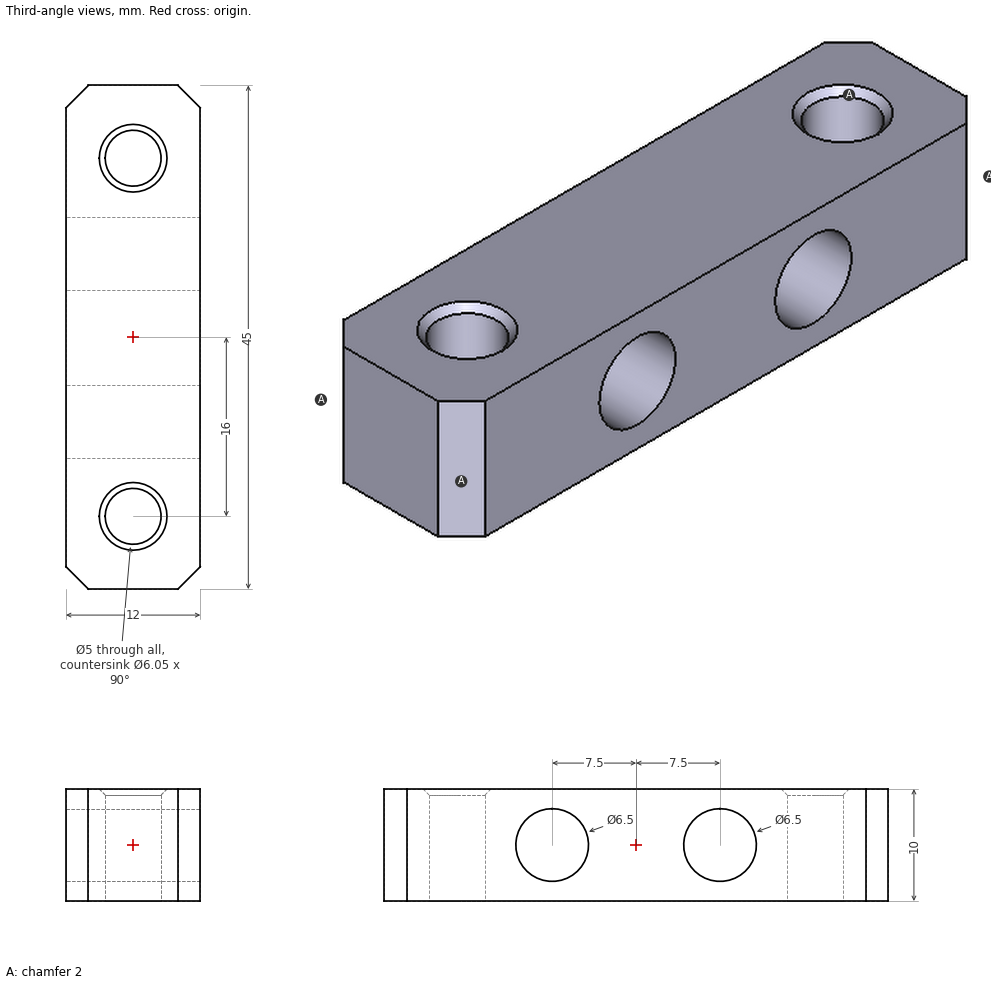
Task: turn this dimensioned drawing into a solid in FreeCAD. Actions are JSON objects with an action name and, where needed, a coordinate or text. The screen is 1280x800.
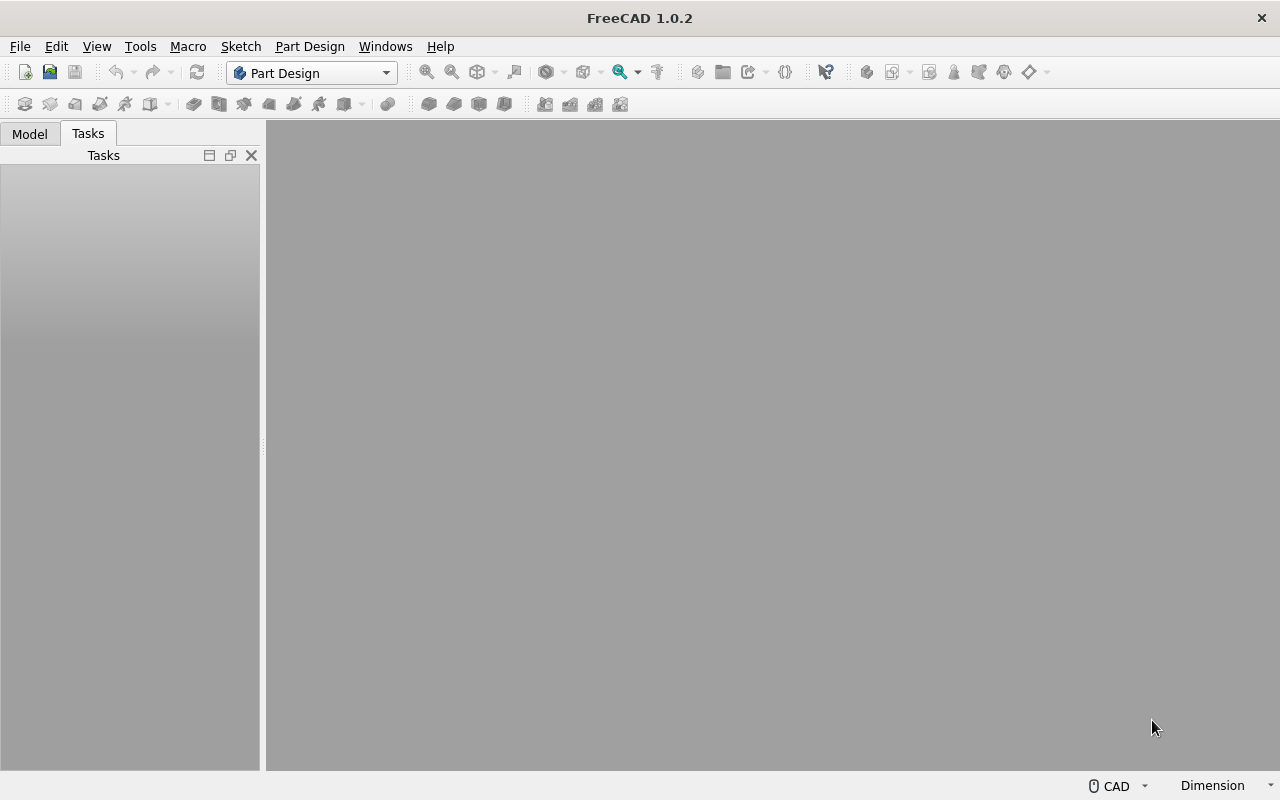
{"action": "left_click", "coordinate": [25, 72]}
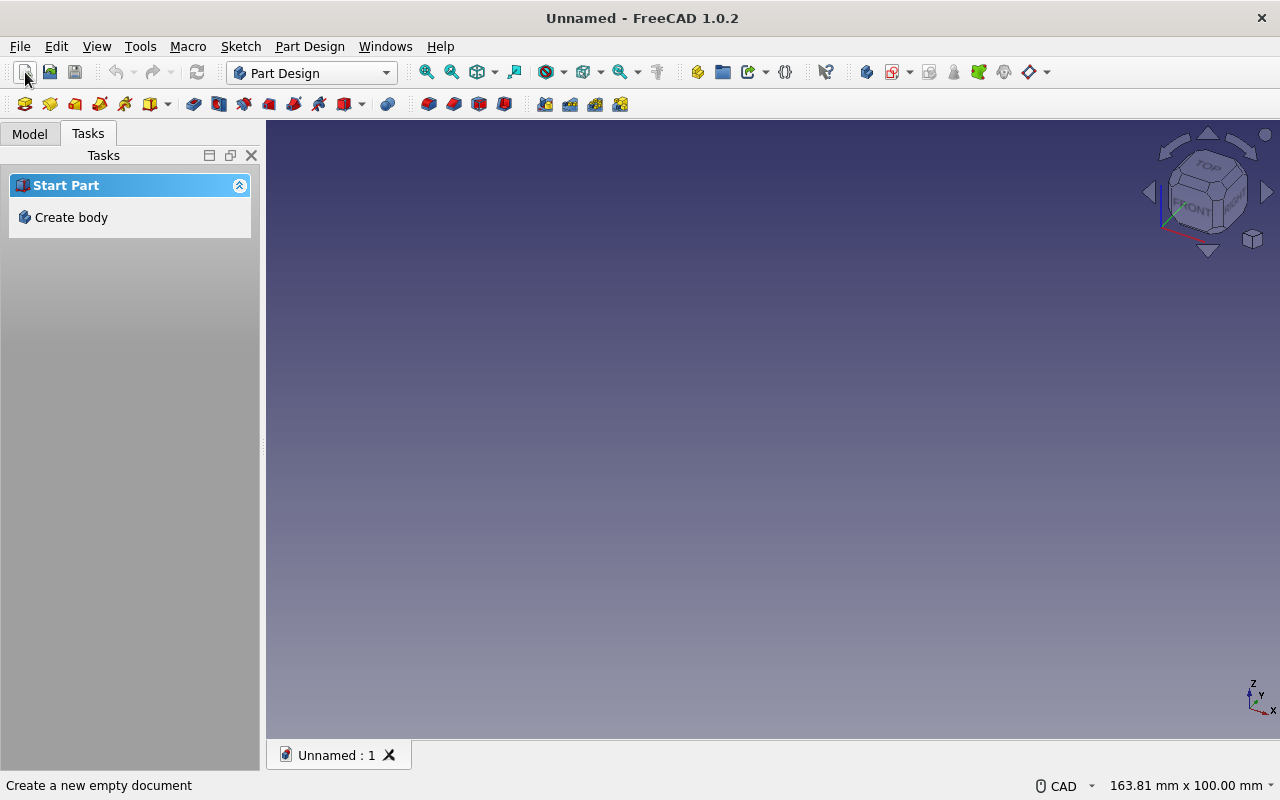
{"action": "left_click", "coordinate": [892, 72]}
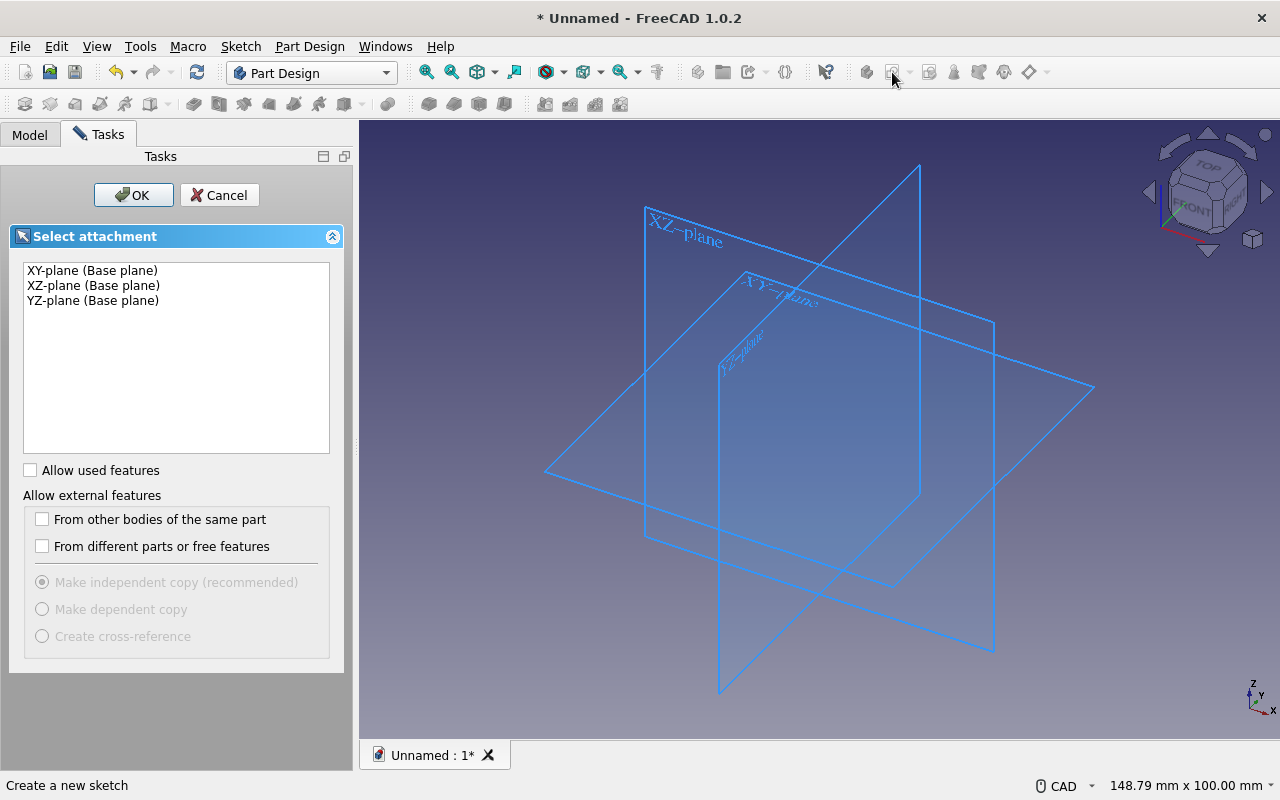
{"action": "left_click", "coordinate": [84, 270]}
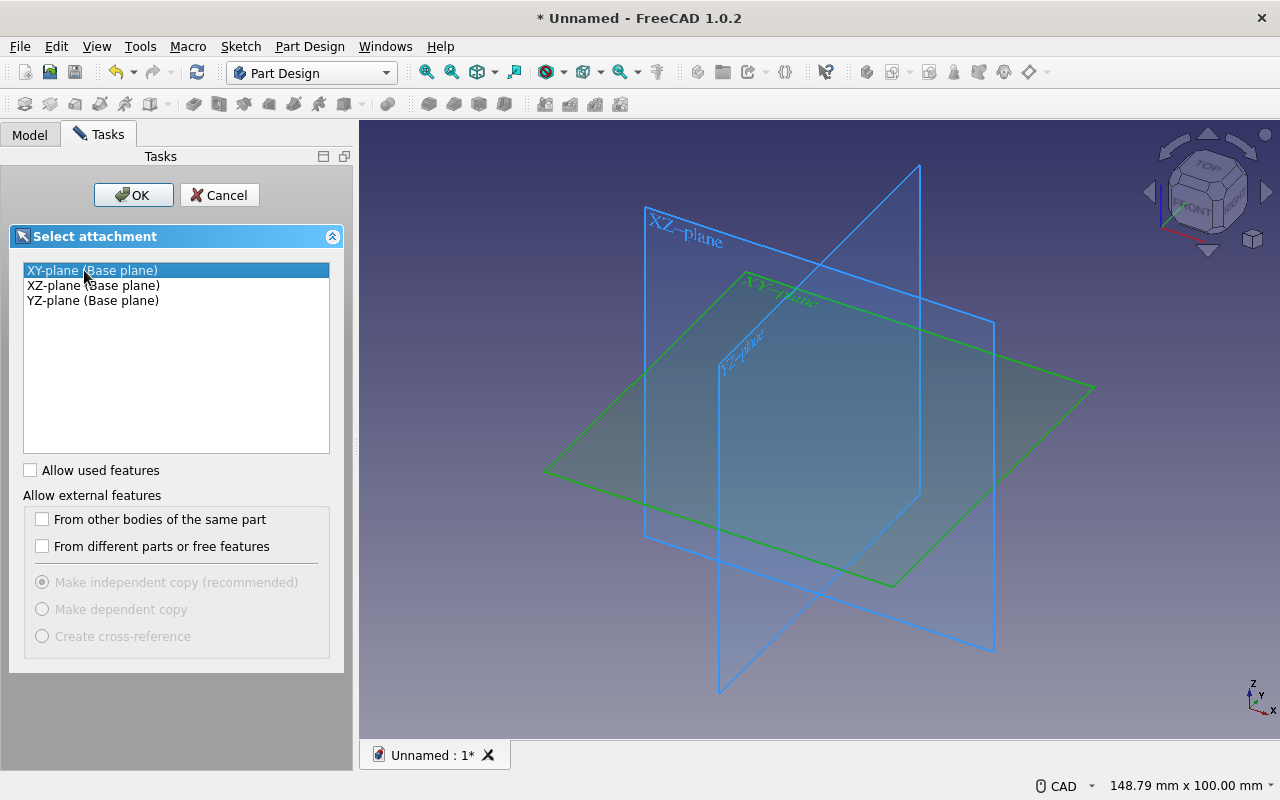
{"action": "left_click", "coordinate": [134, 195]}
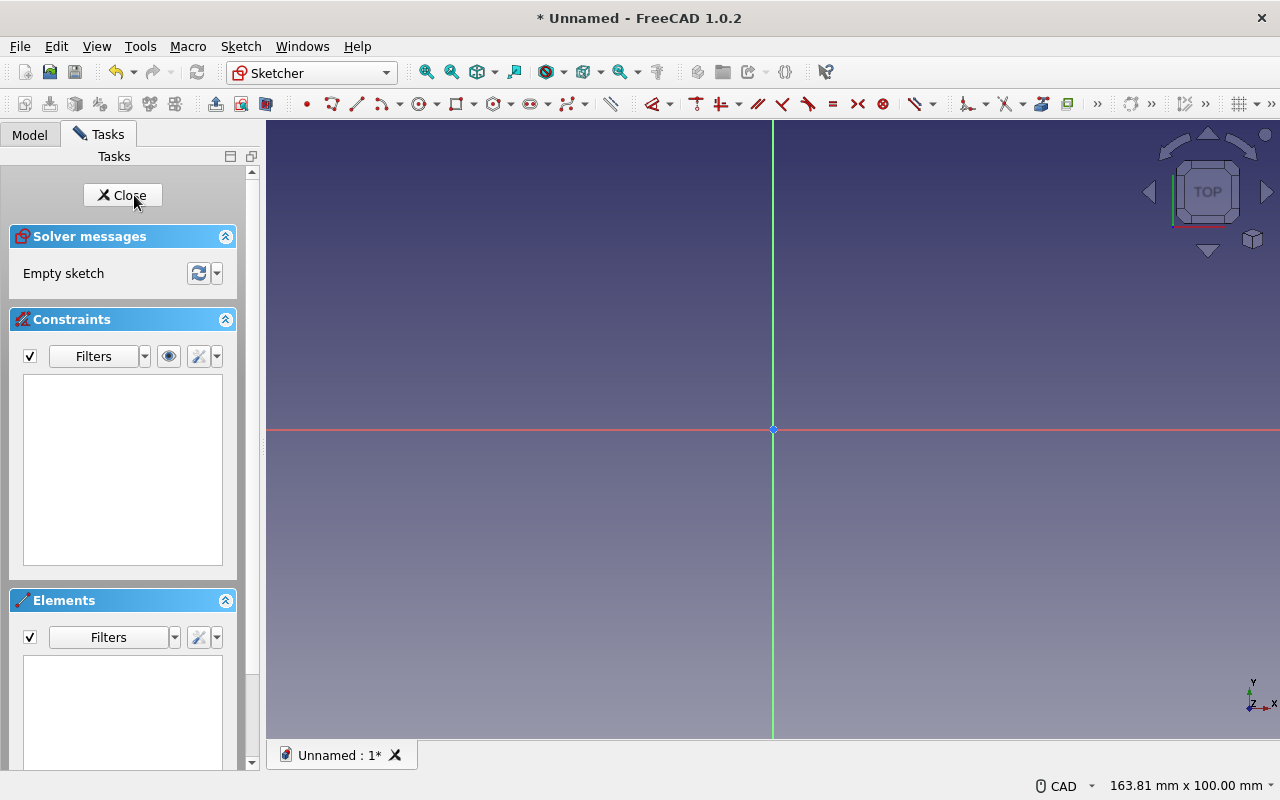
{"action": "scroll", "coordinate": [912, 429], "scroll_direction": "up", "scroll_amount": 2}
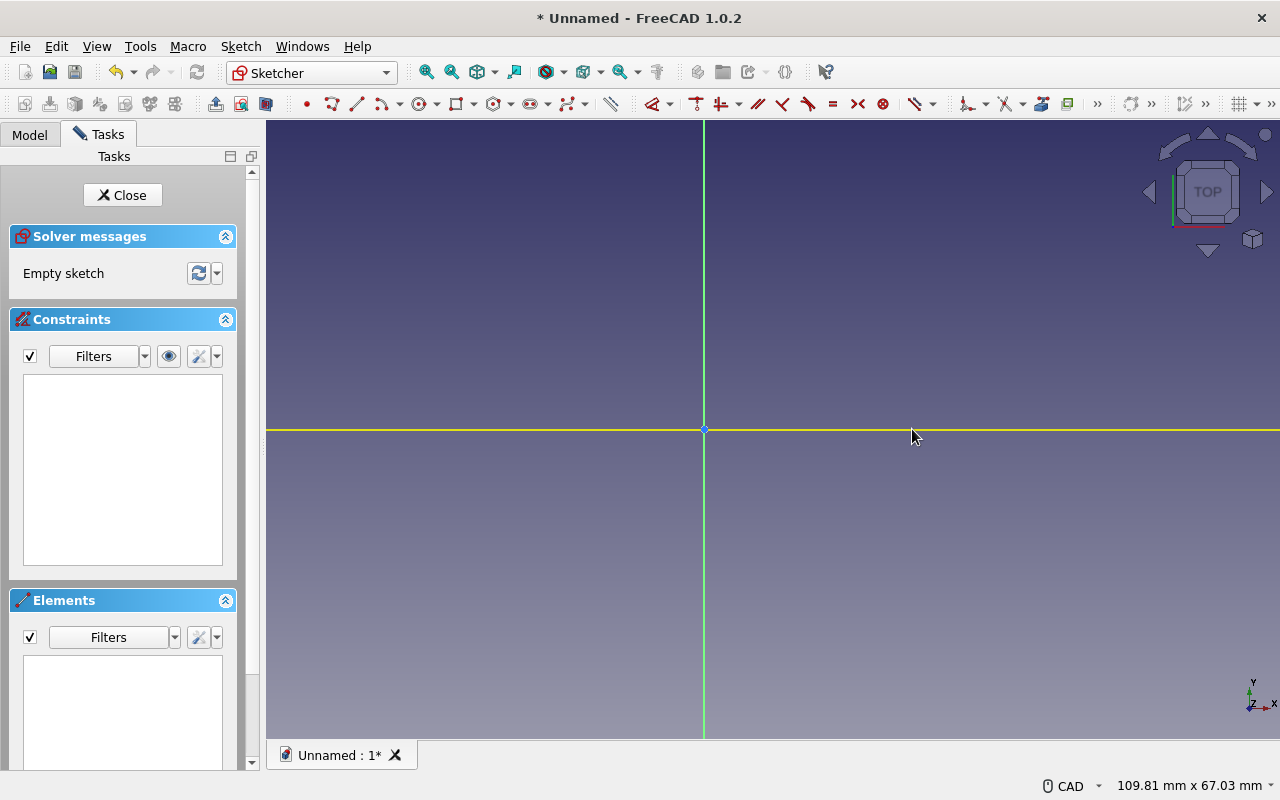
{"action": "key", "text": "g v"}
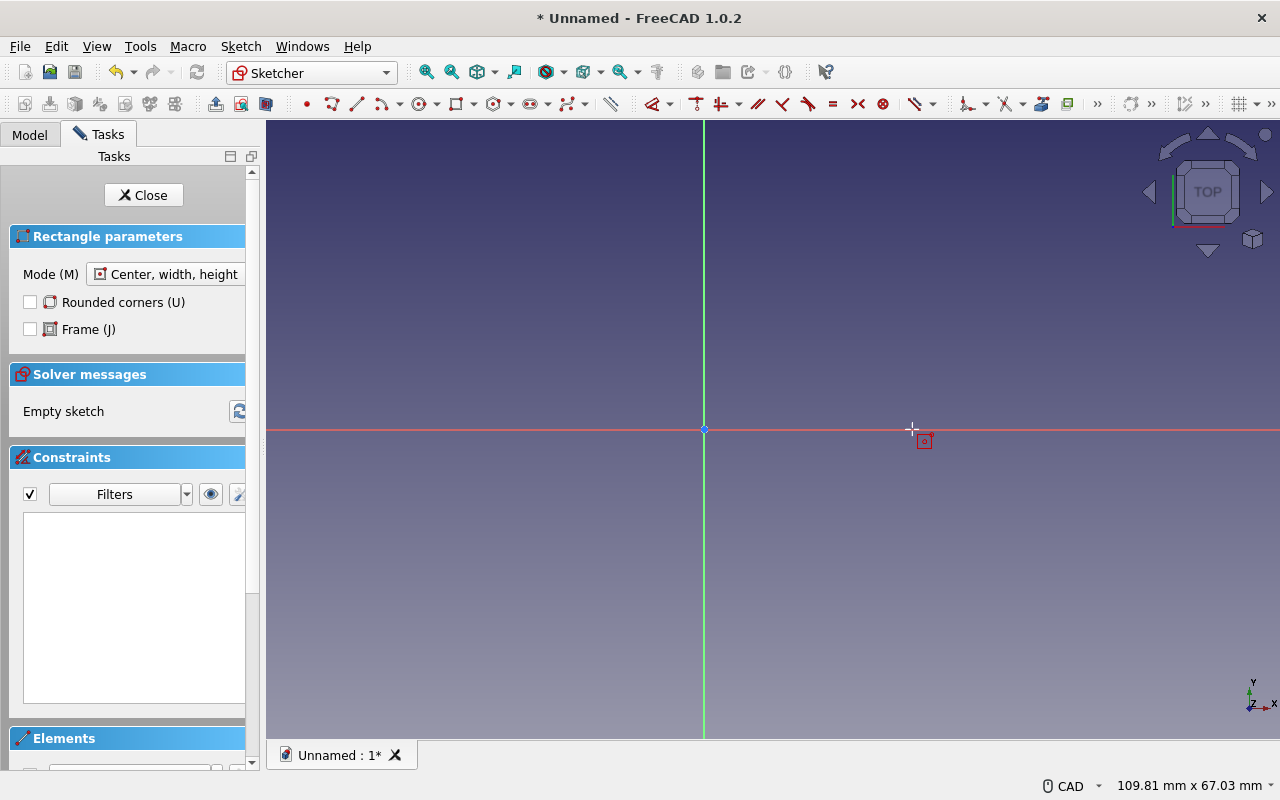
{"action": "left_click", "coordinate": [704, 430]}
{"action": "mouse_move", "coordinate": [760, 222]}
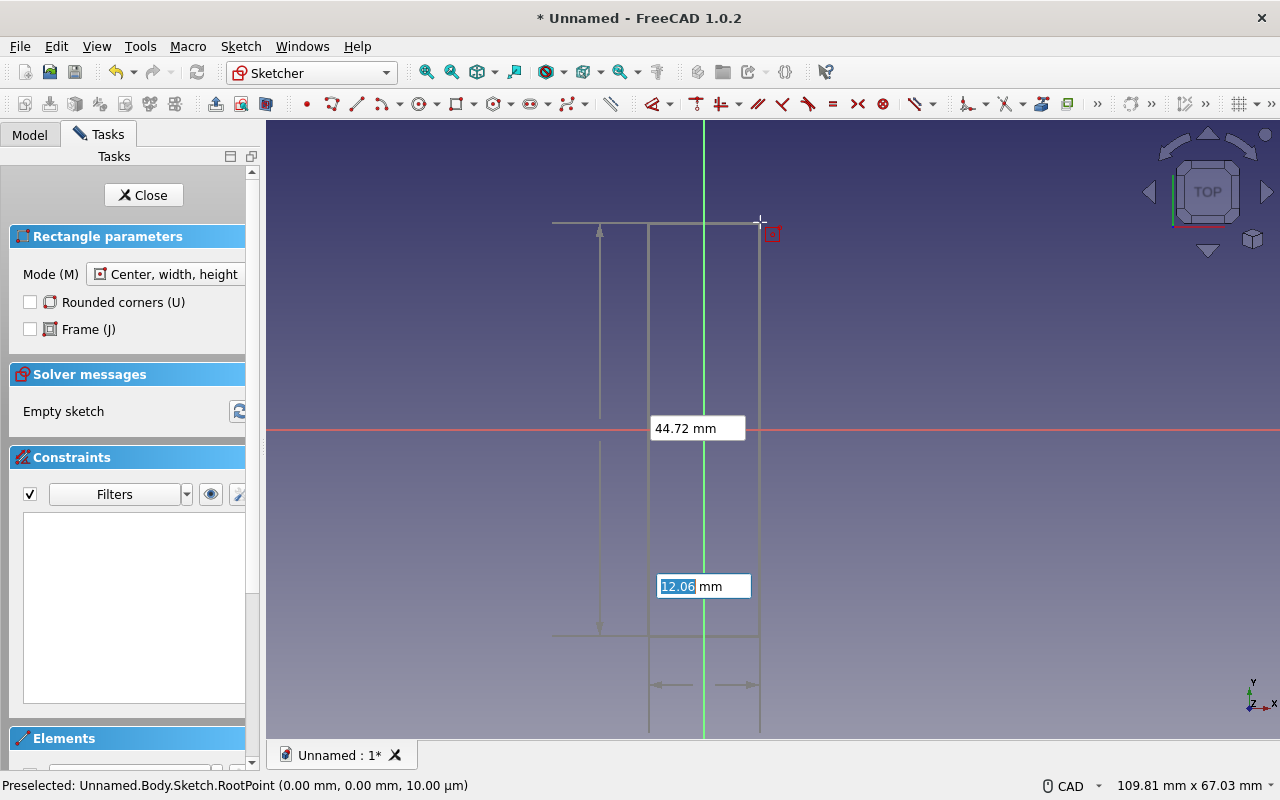
{"action": "type", "text": "12"}
{"action": "key", "text": "Tab"}
{"action": "type", "text": "45"}
{"action": "key", "text": "Return"}
{"action": "key", "text": "Escape"}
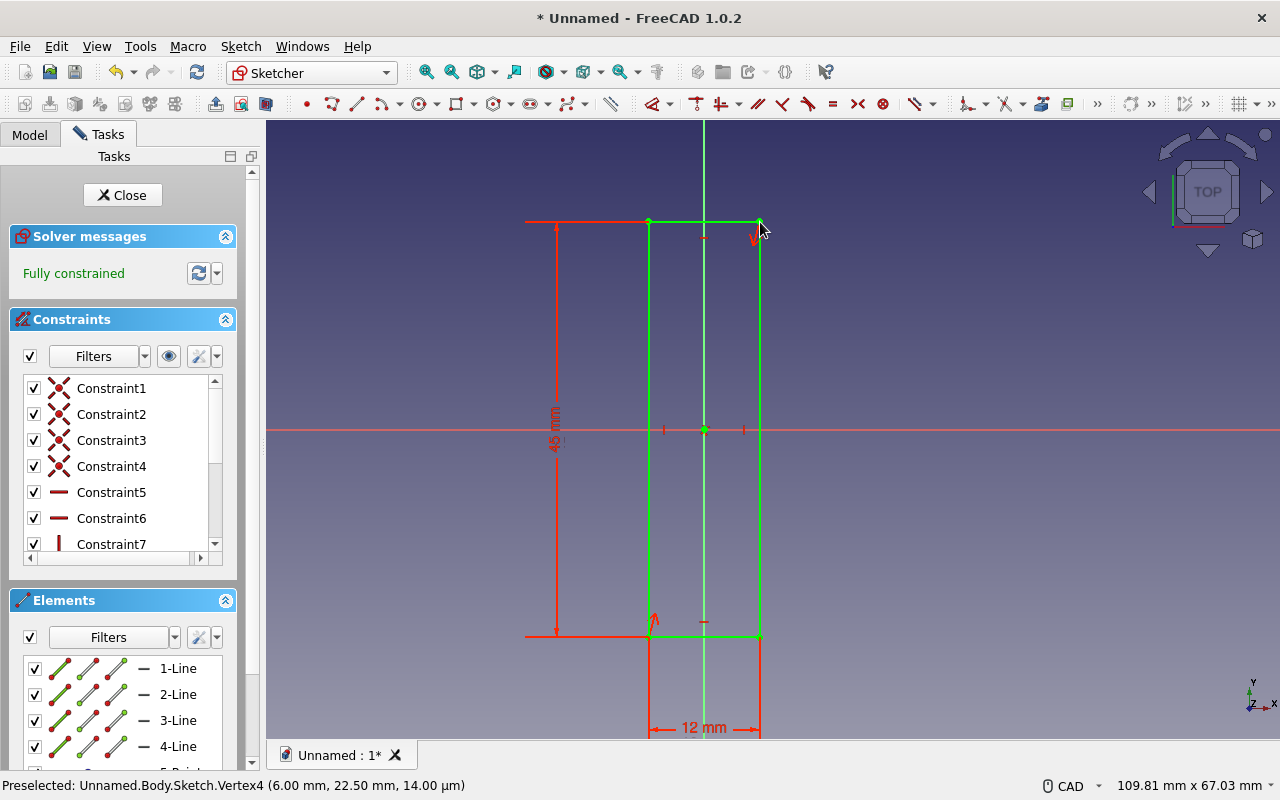
{"action": "left_click", "coordinate": [123, 195]}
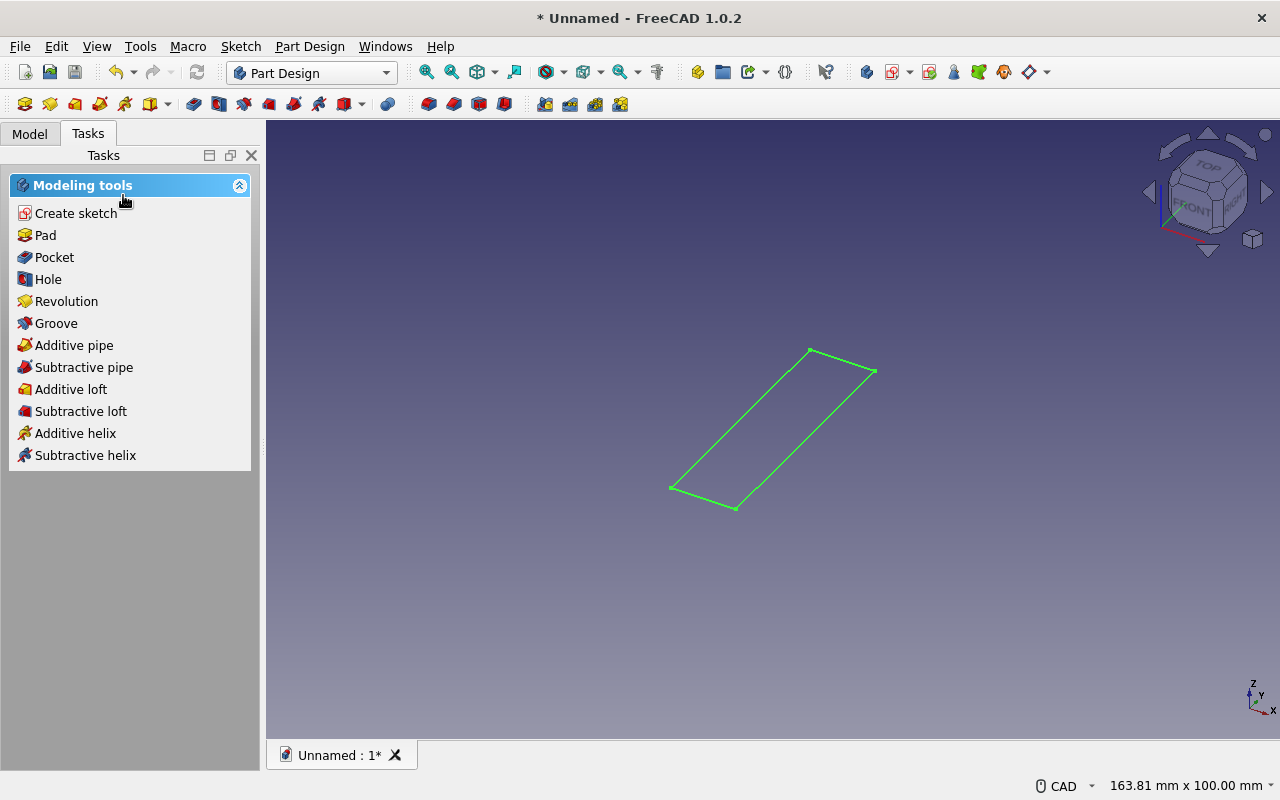
{"action": "left_click", "coordinate": [25, 104]}